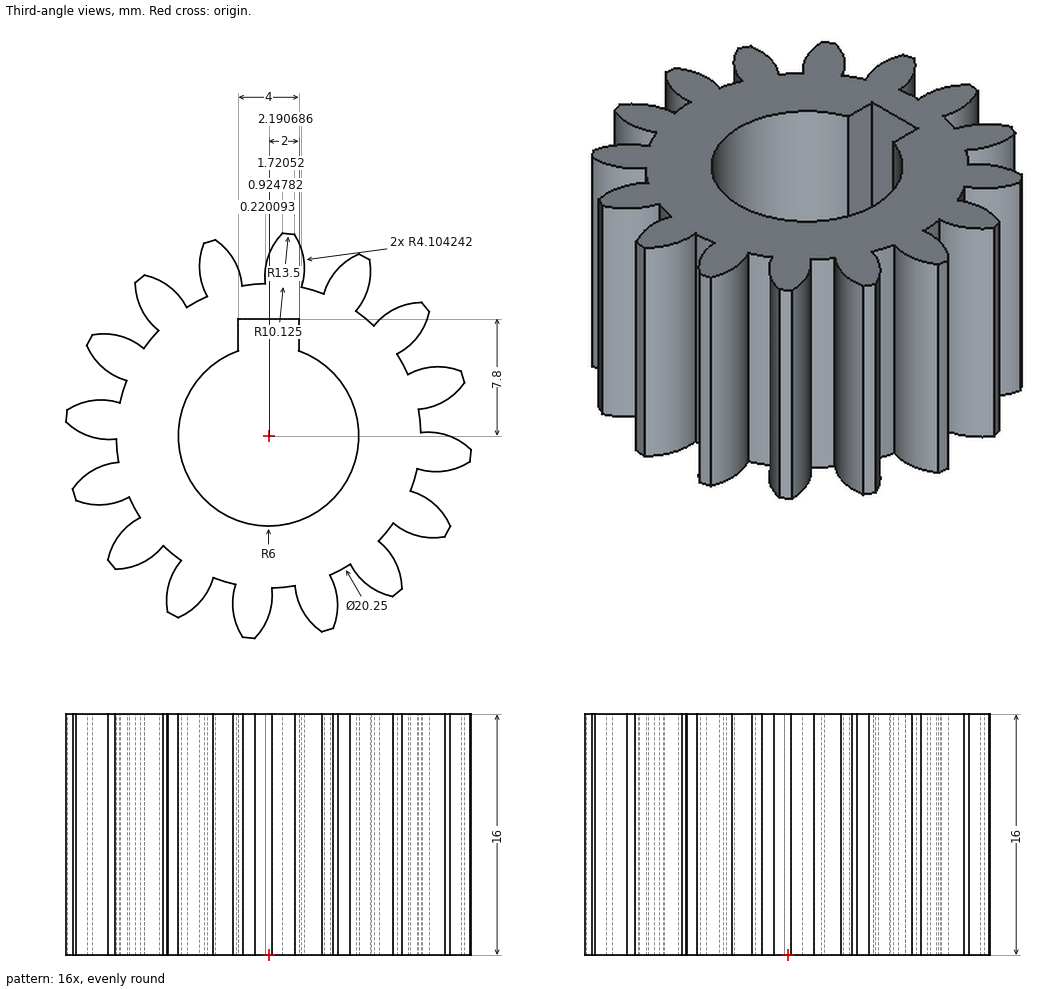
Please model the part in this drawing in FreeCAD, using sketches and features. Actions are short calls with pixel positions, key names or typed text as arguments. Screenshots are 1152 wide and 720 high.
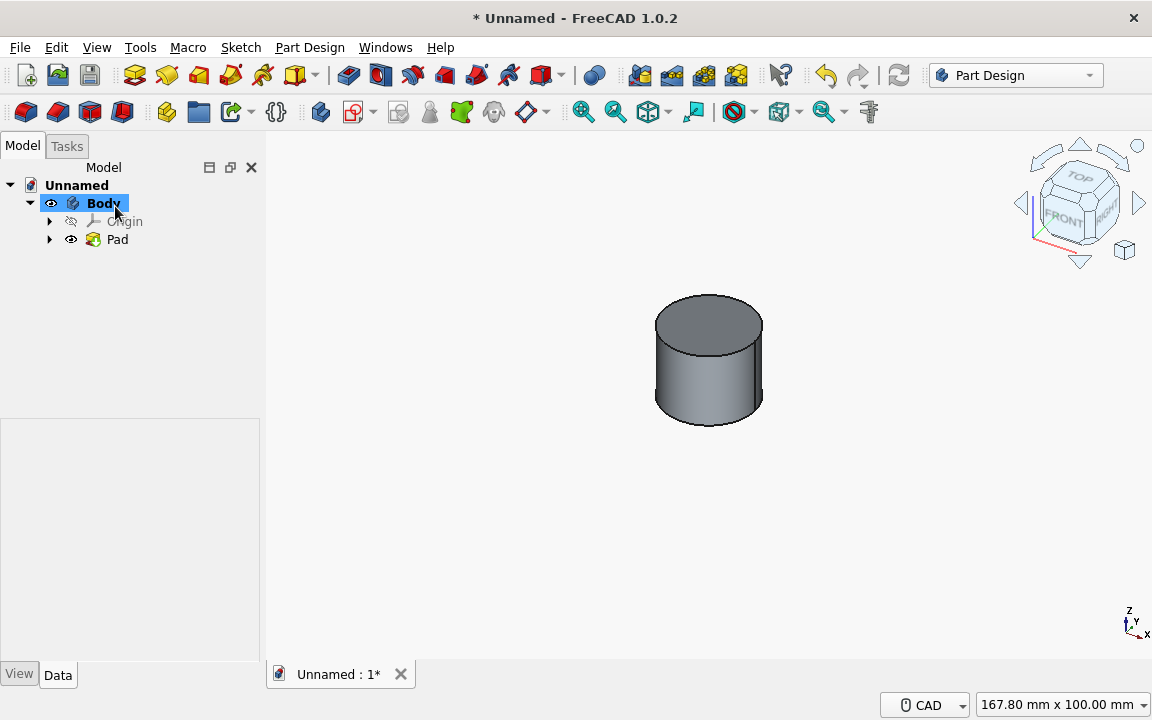
click(584, 112)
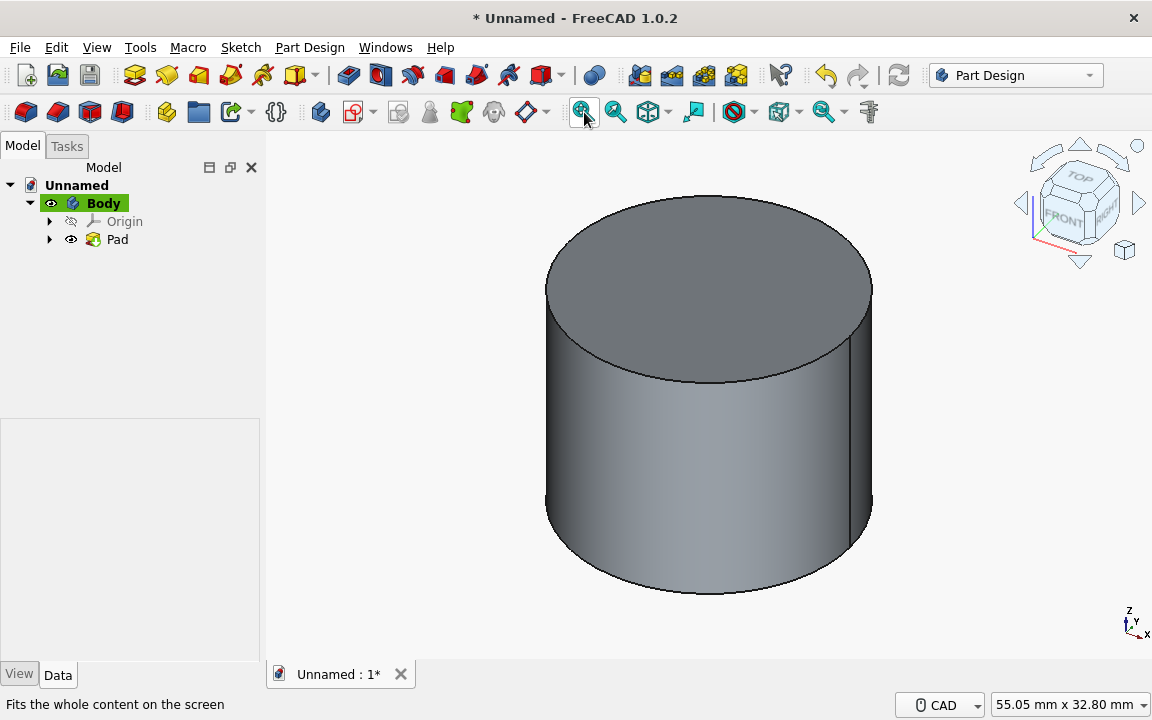
click(354, 112)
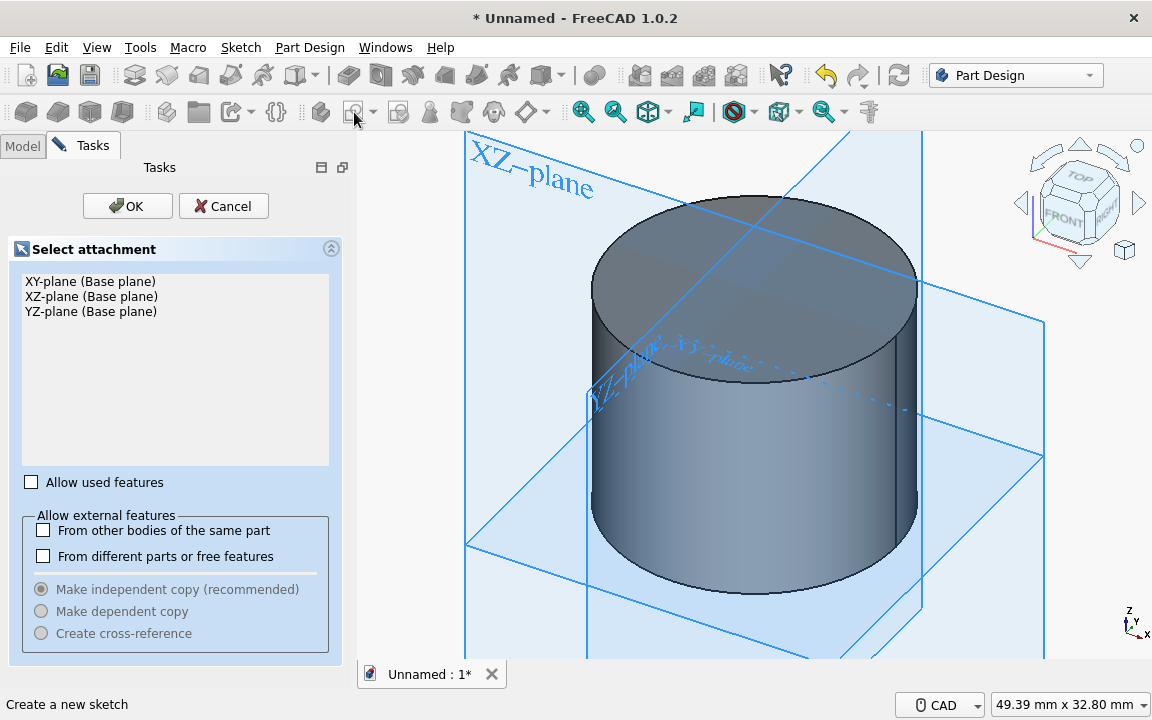
click(82, 282)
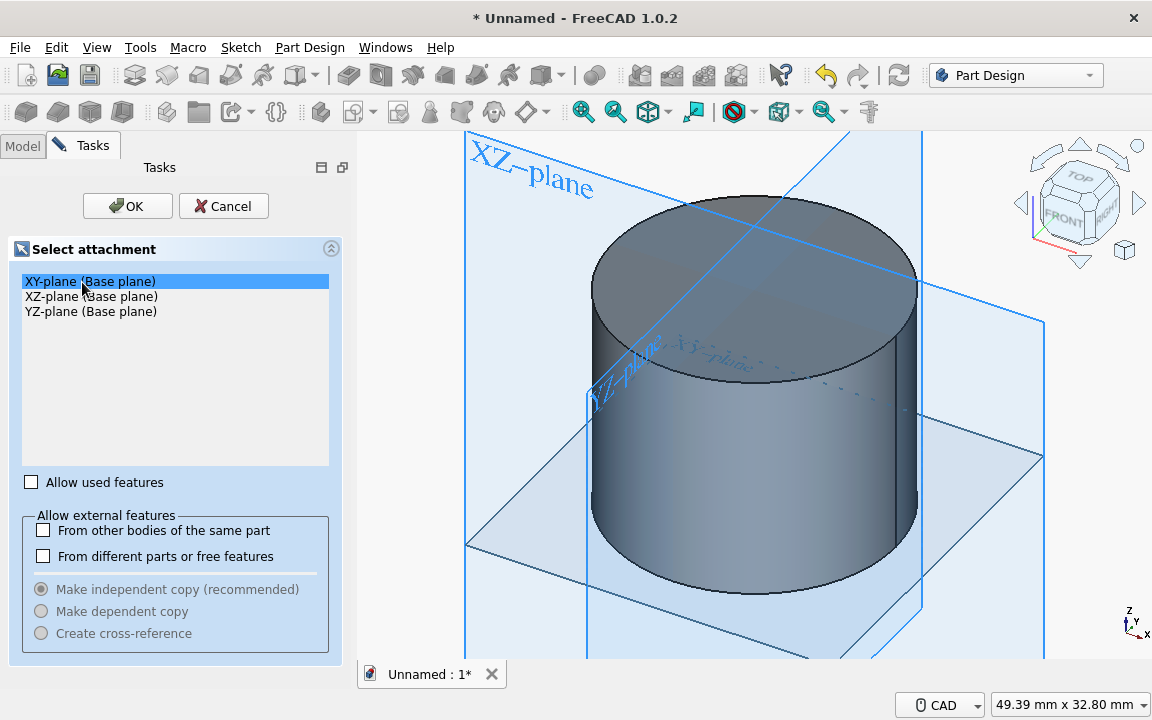
click(128, 206)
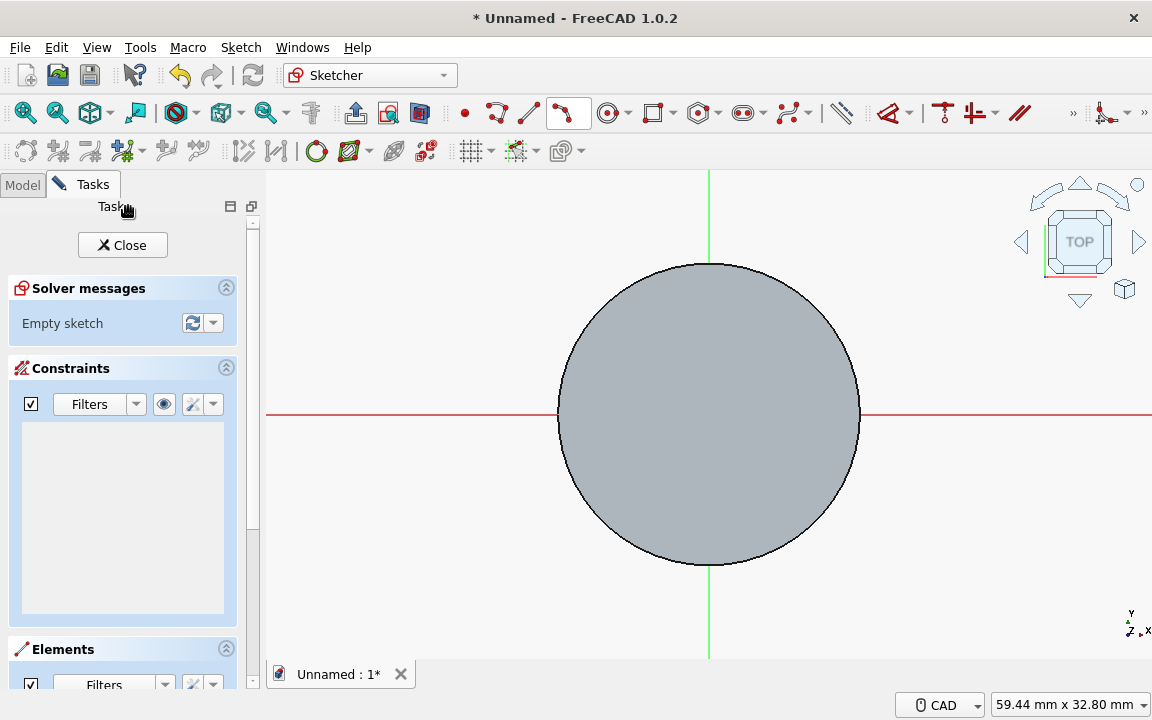
click(420, 114)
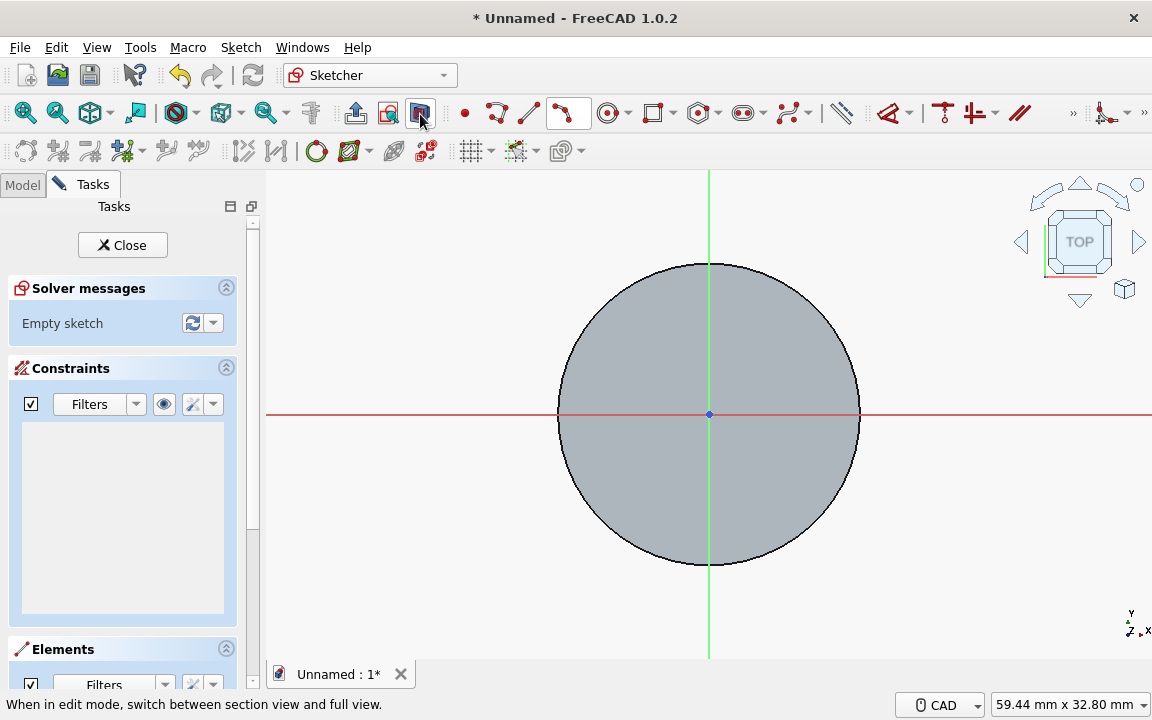
scroll(742, 206, up, 9)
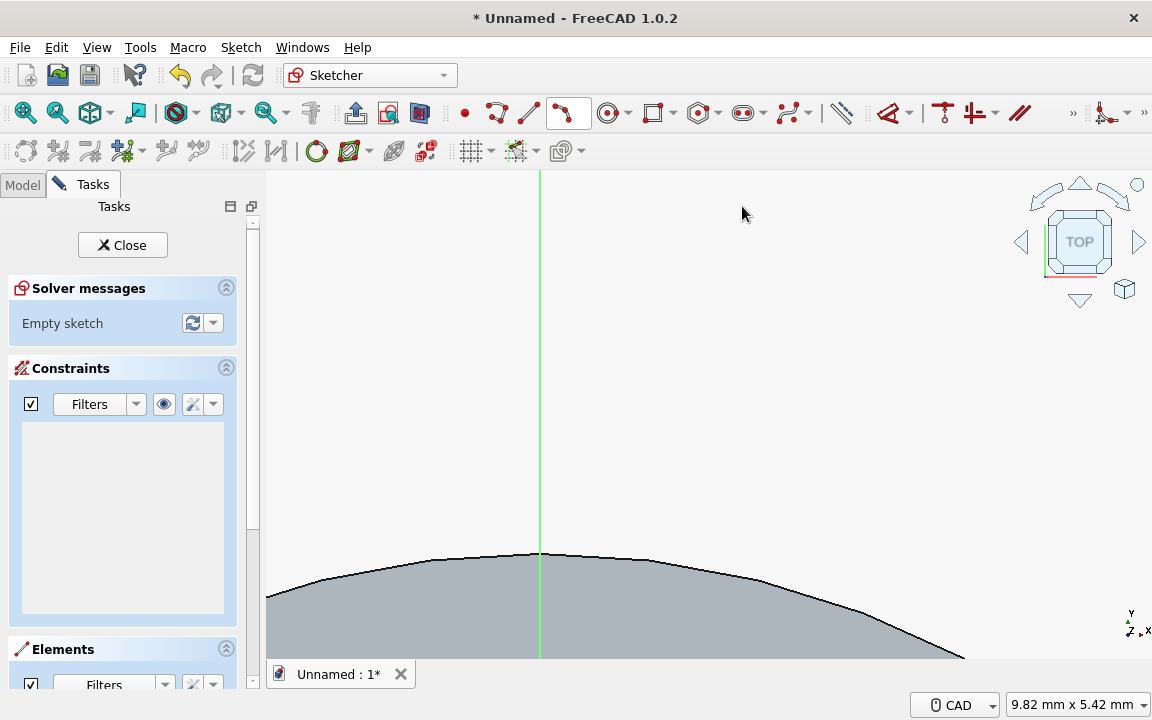
click(562, 114)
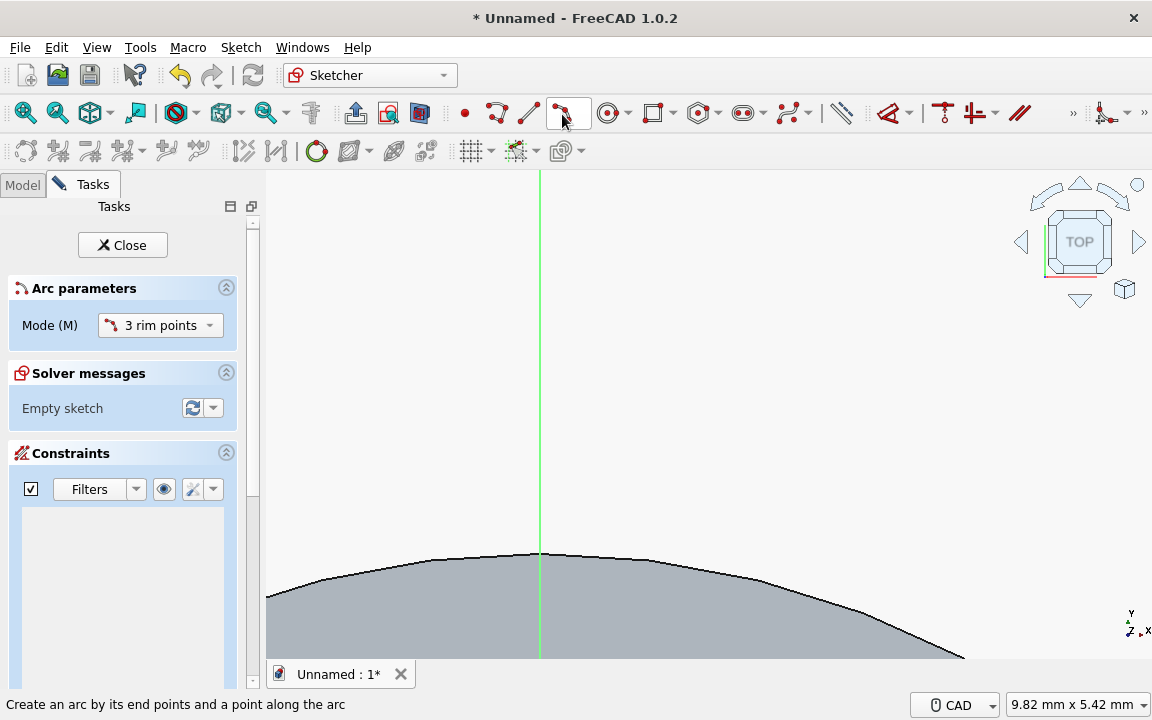
click(520, 554)
click(737, 576)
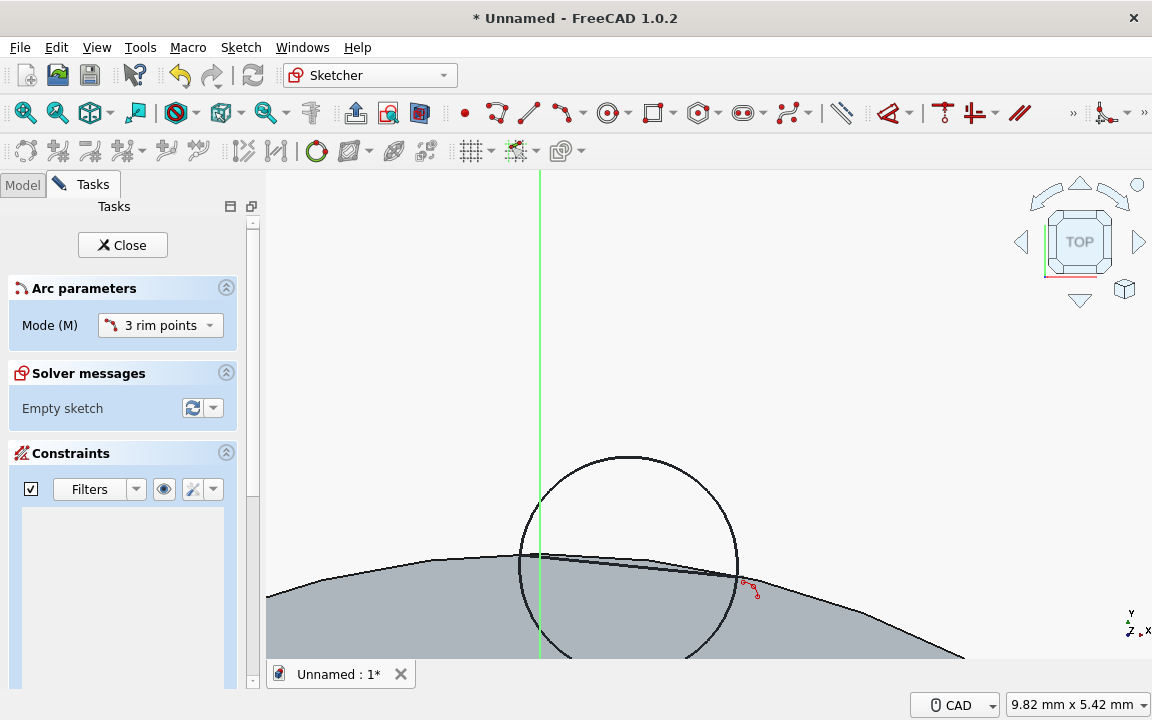
scroll(629, 558, up, 5)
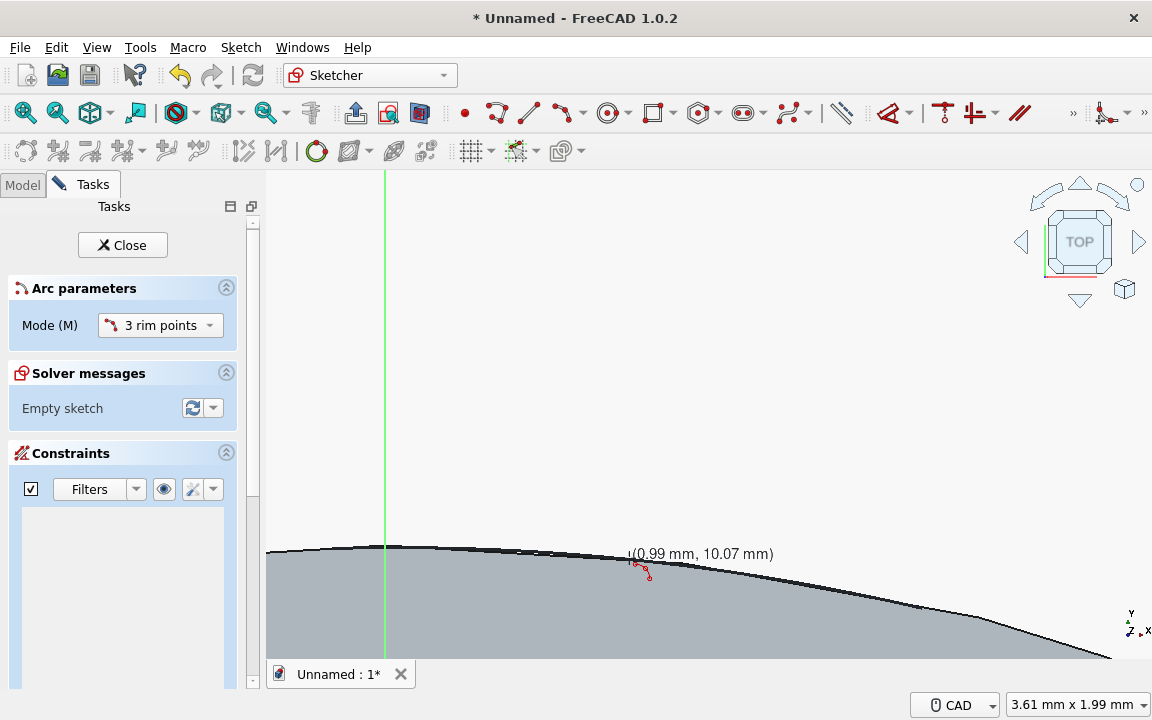
click(629, 557)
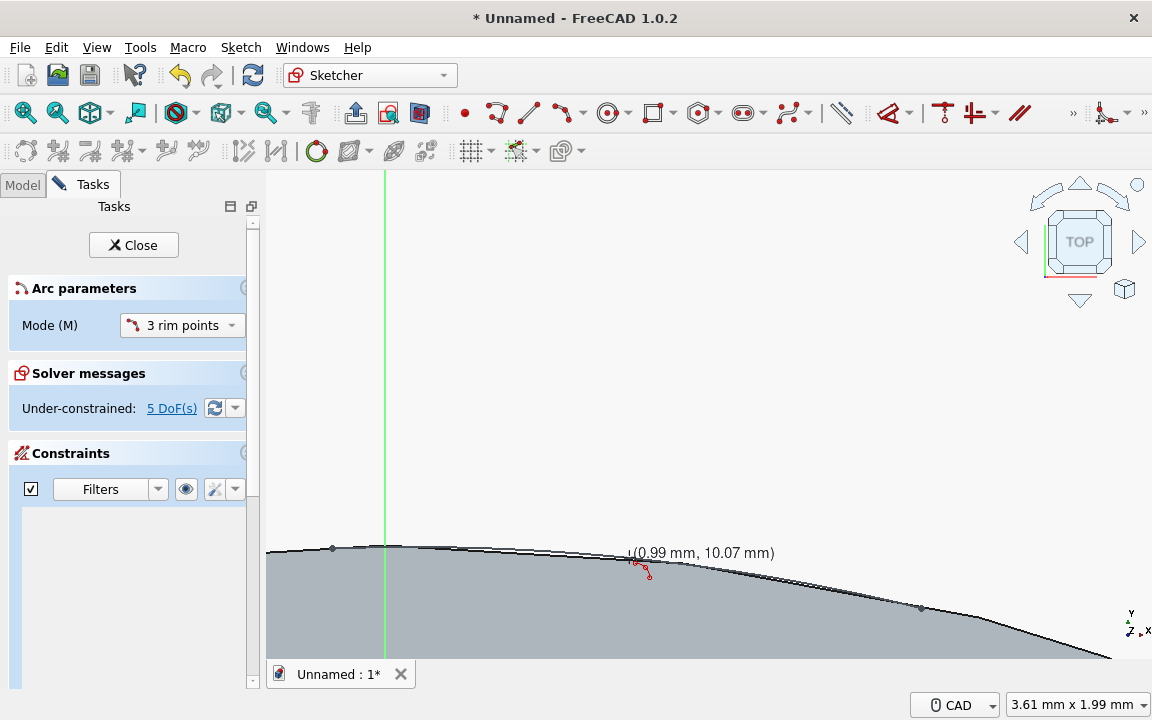
click(922, 608)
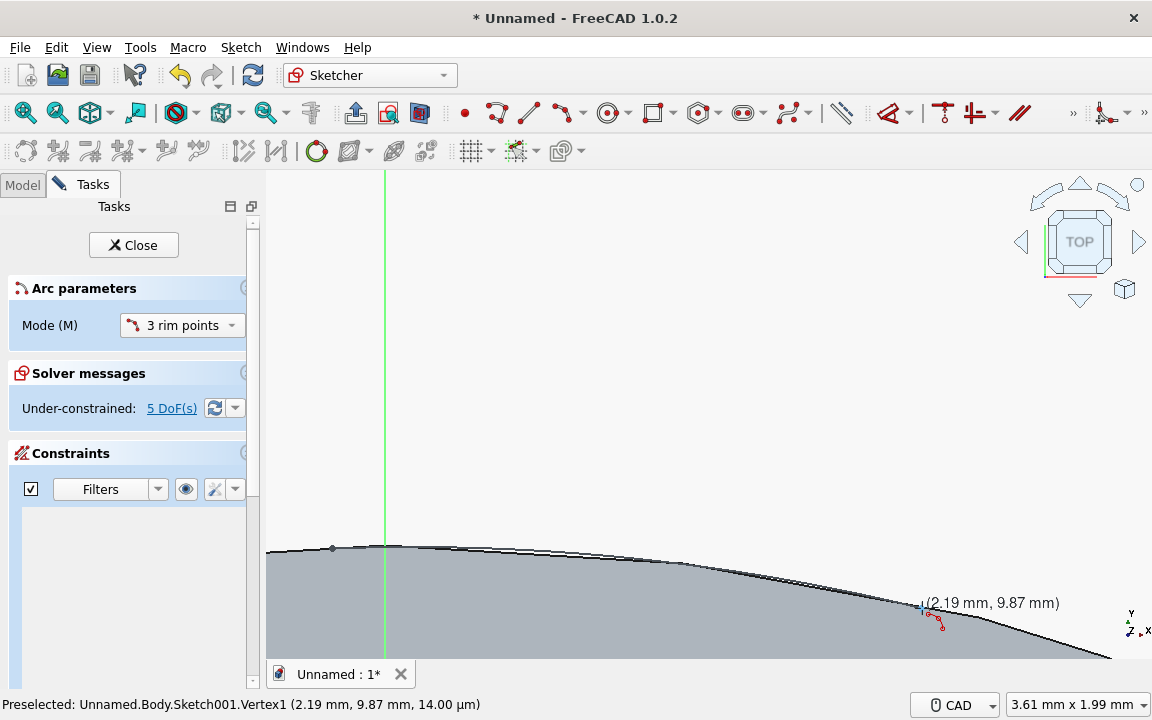
scroll(637, 560, down, 5)